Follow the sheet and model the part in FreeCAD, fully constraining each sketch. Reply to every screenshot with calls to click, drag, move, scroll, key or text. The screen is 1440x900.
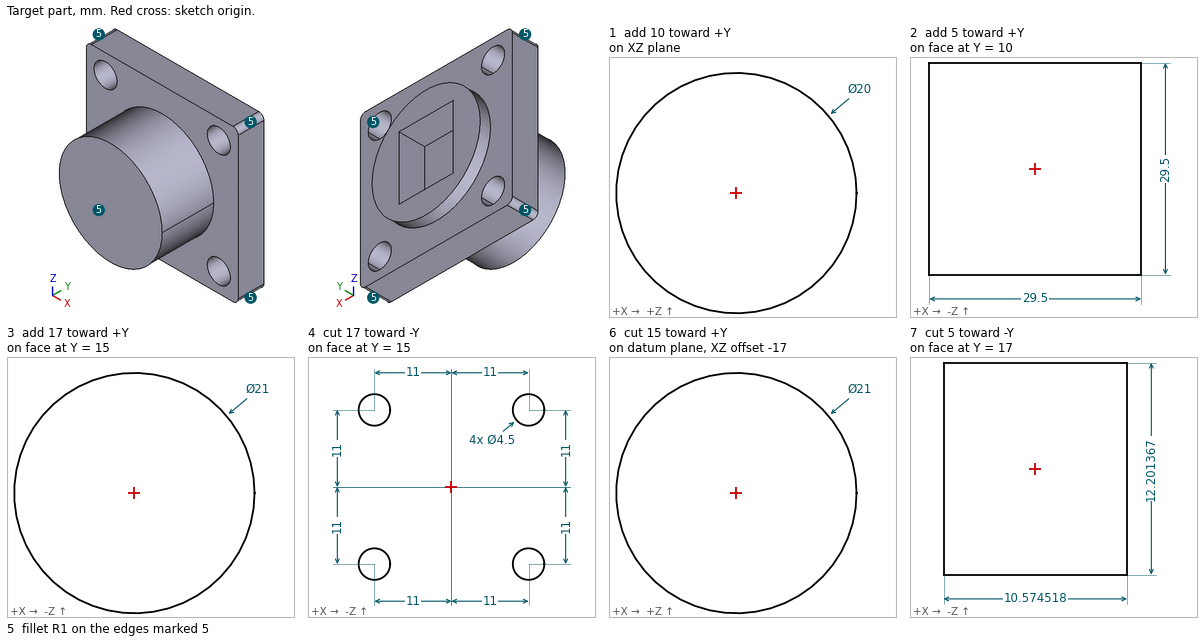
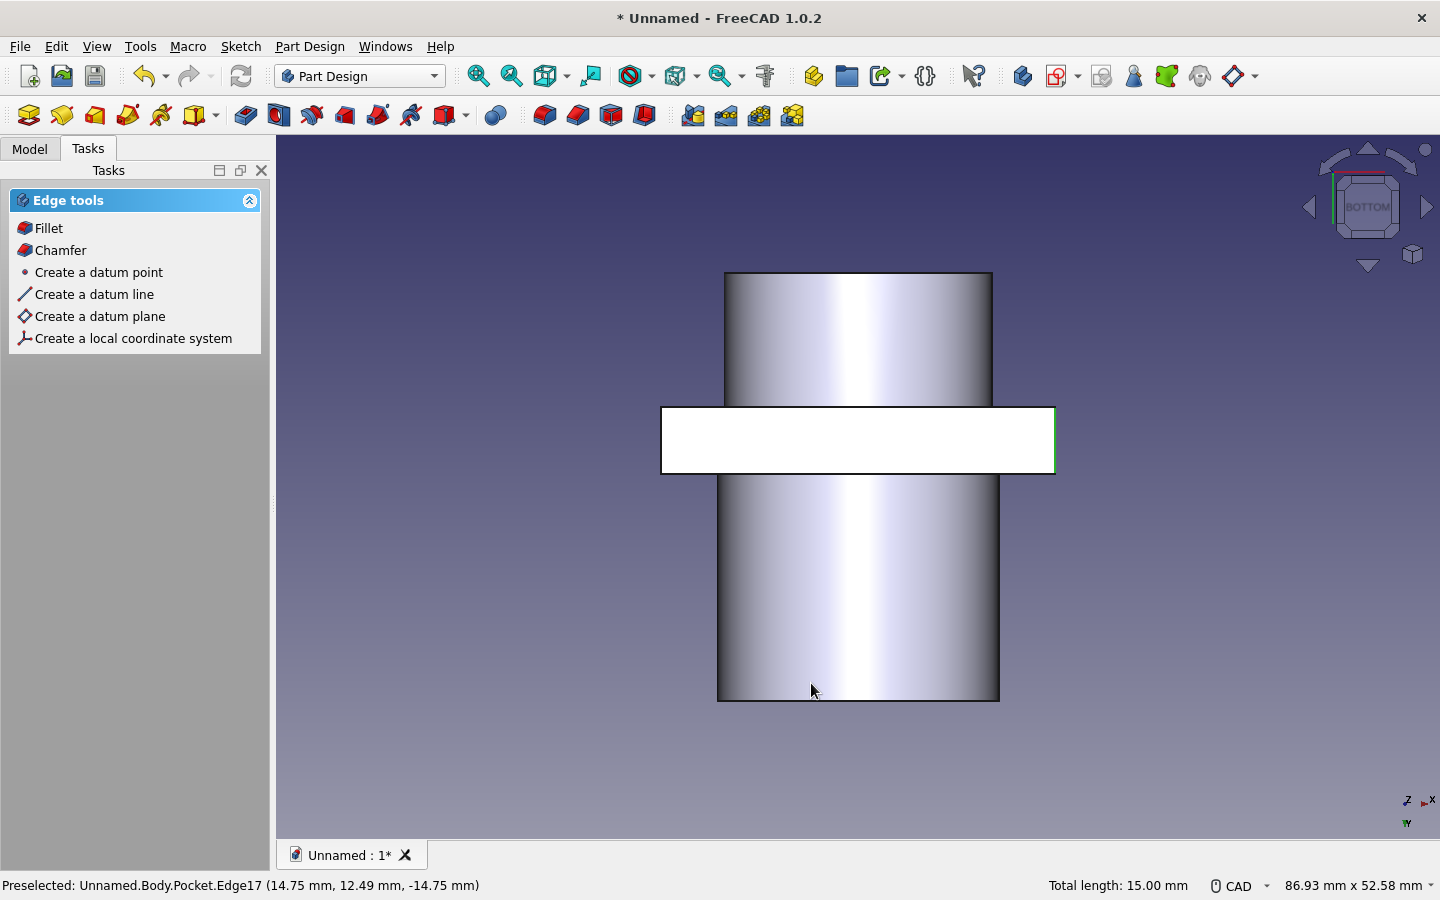
click(661, 439, ctrl)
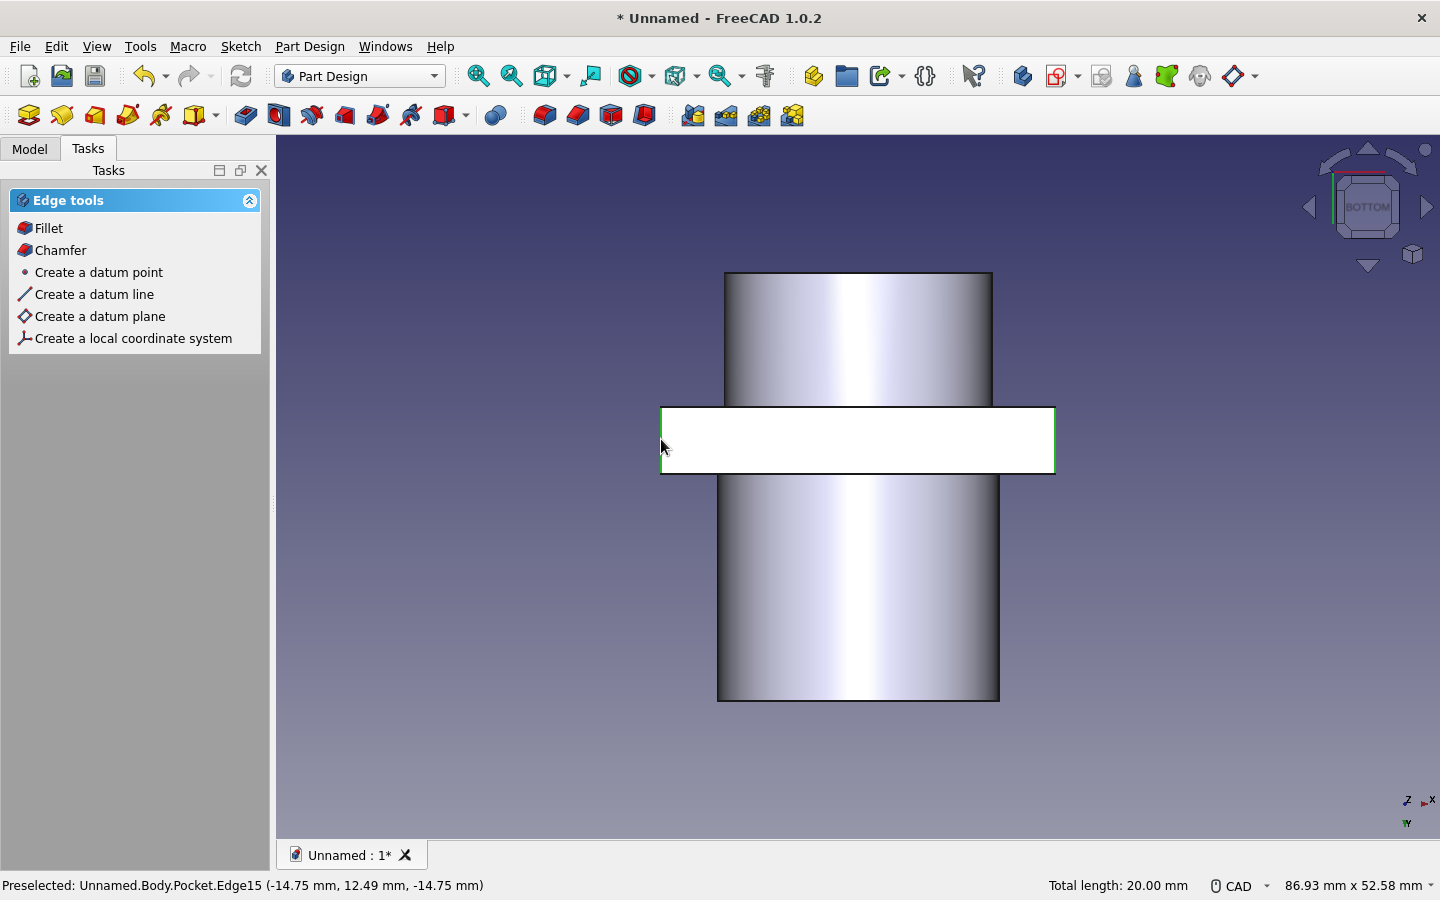
click(545, 116)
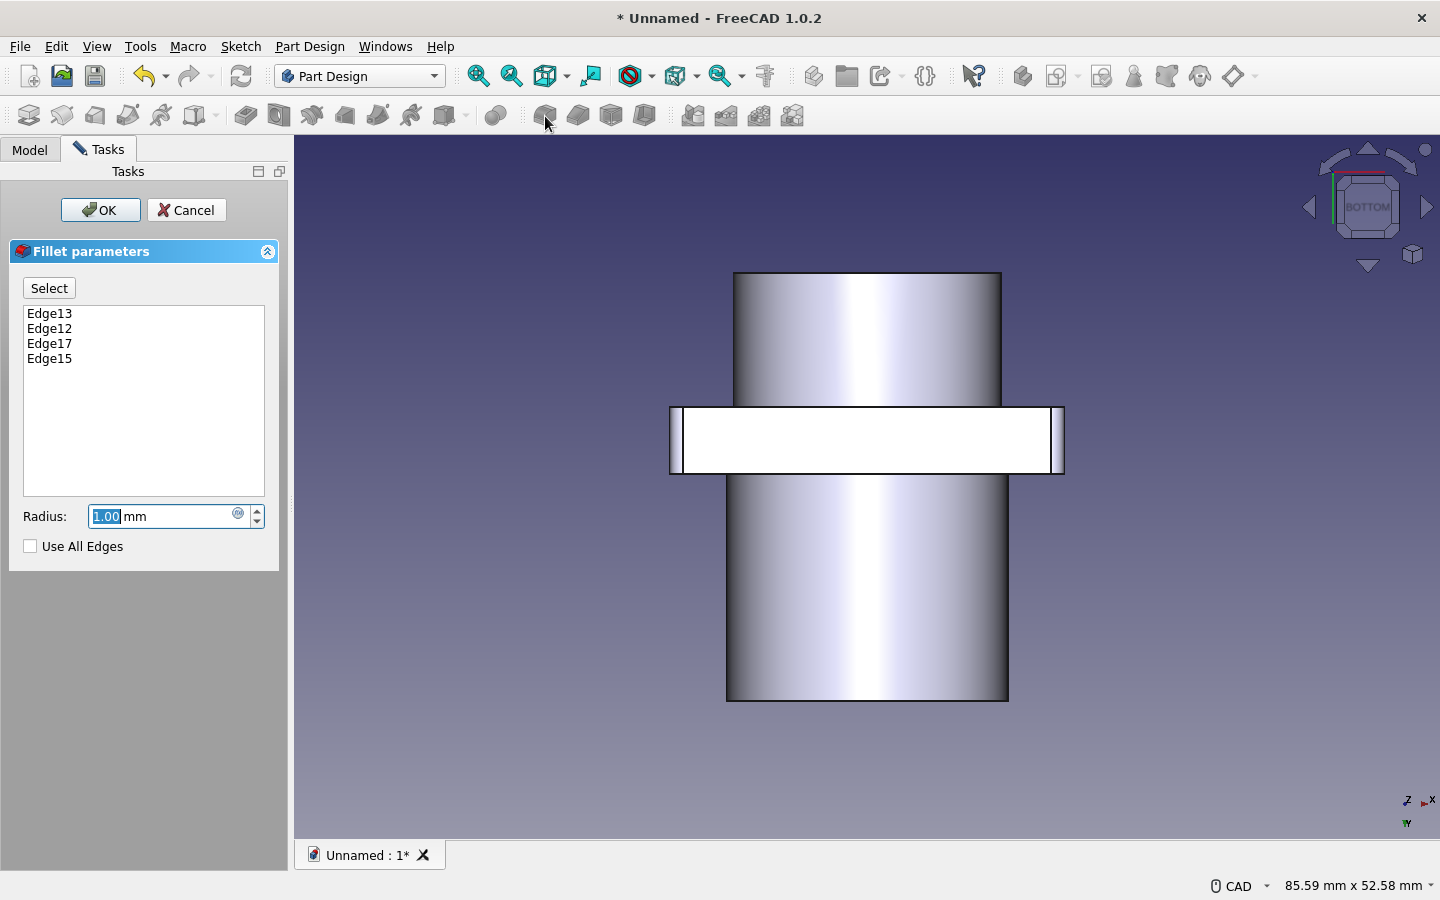
text(1)
key(Tab)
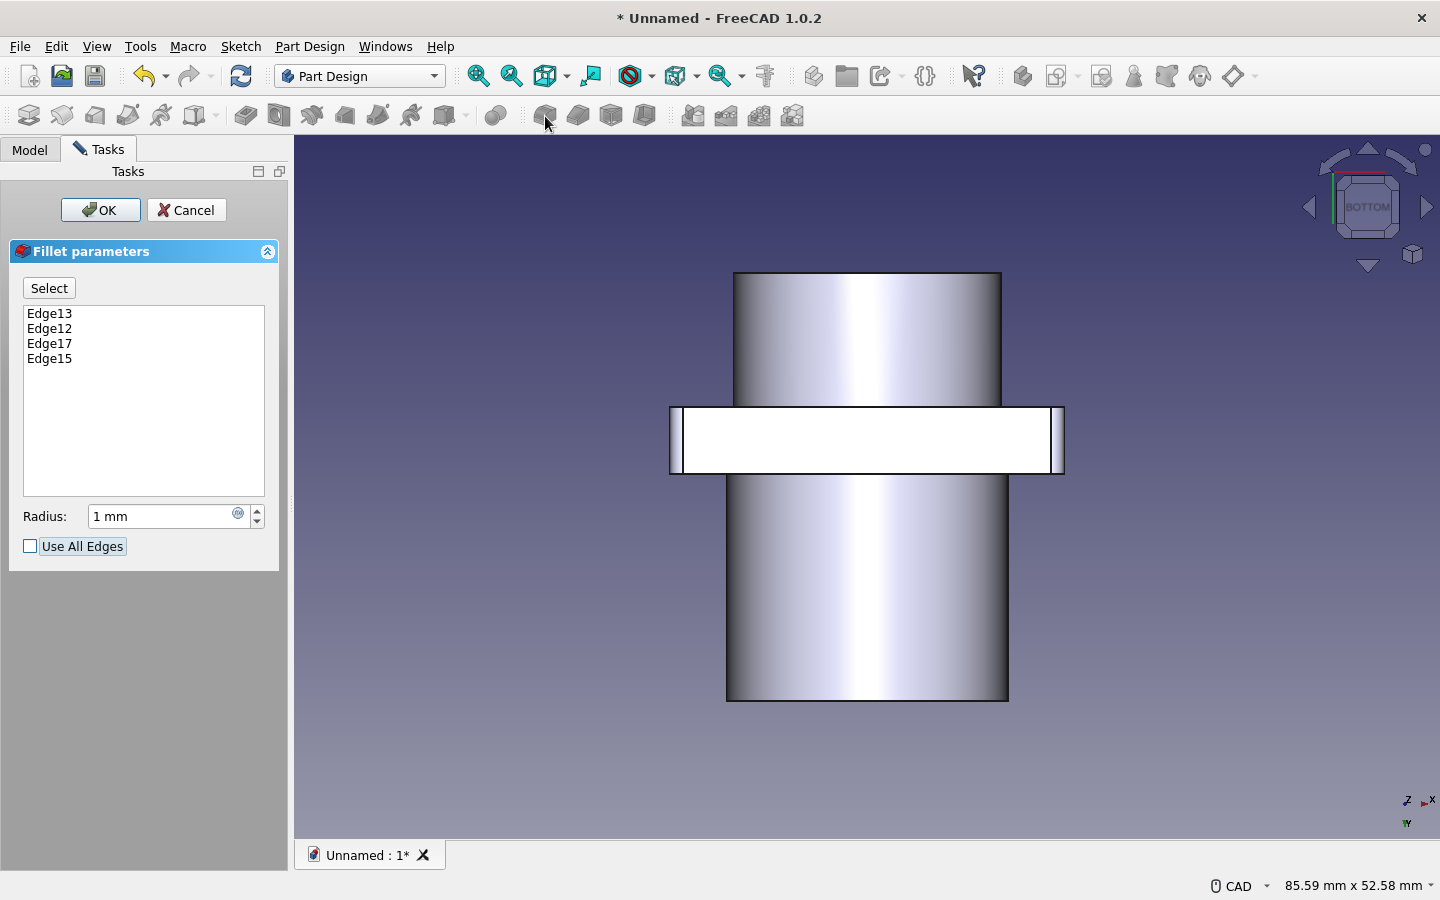
click(101, 210)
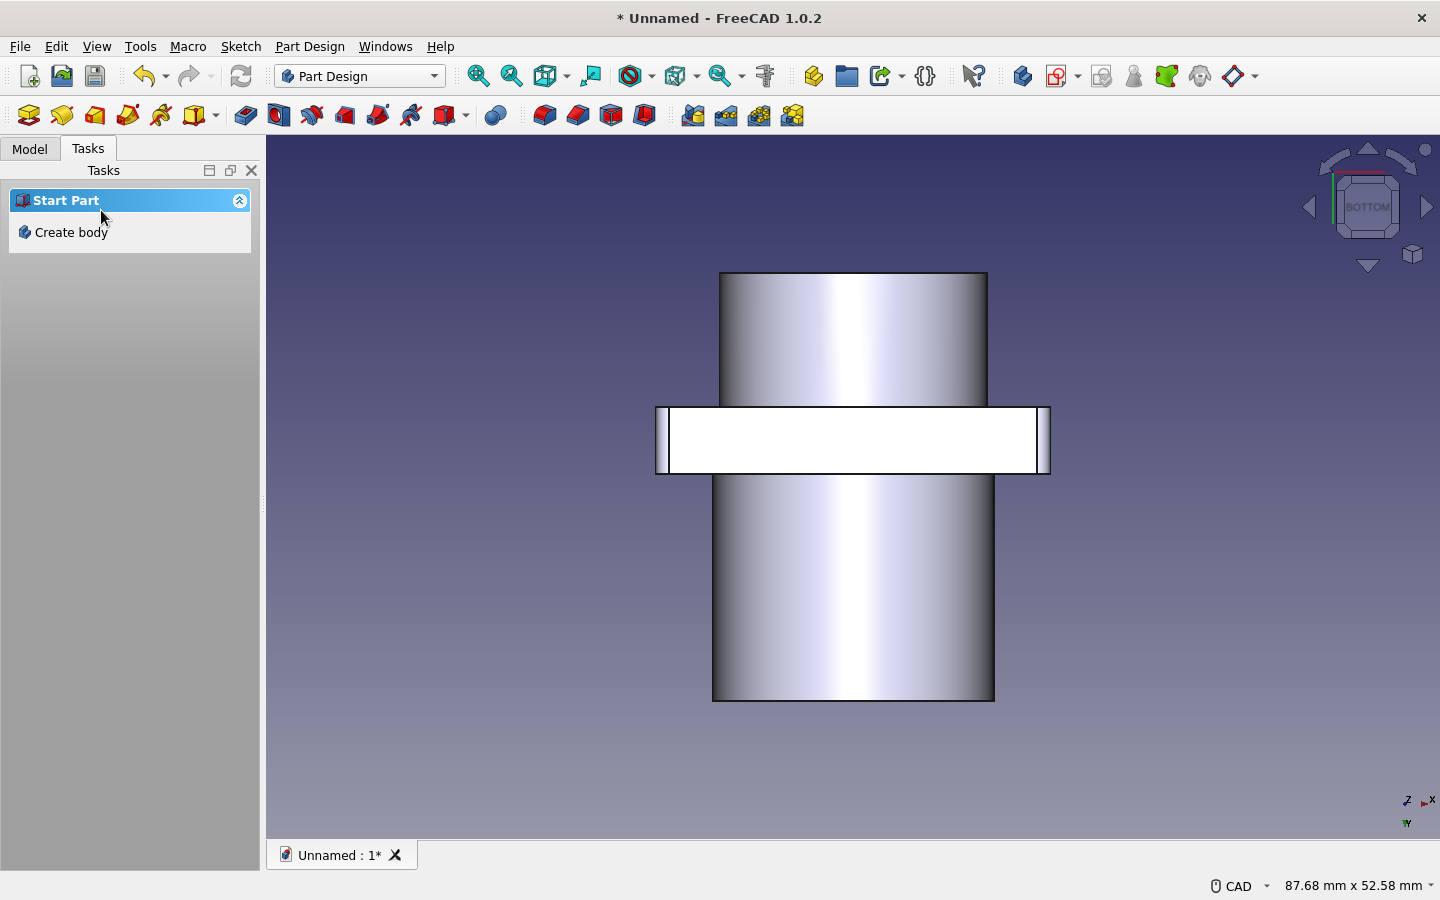
click(30, 148)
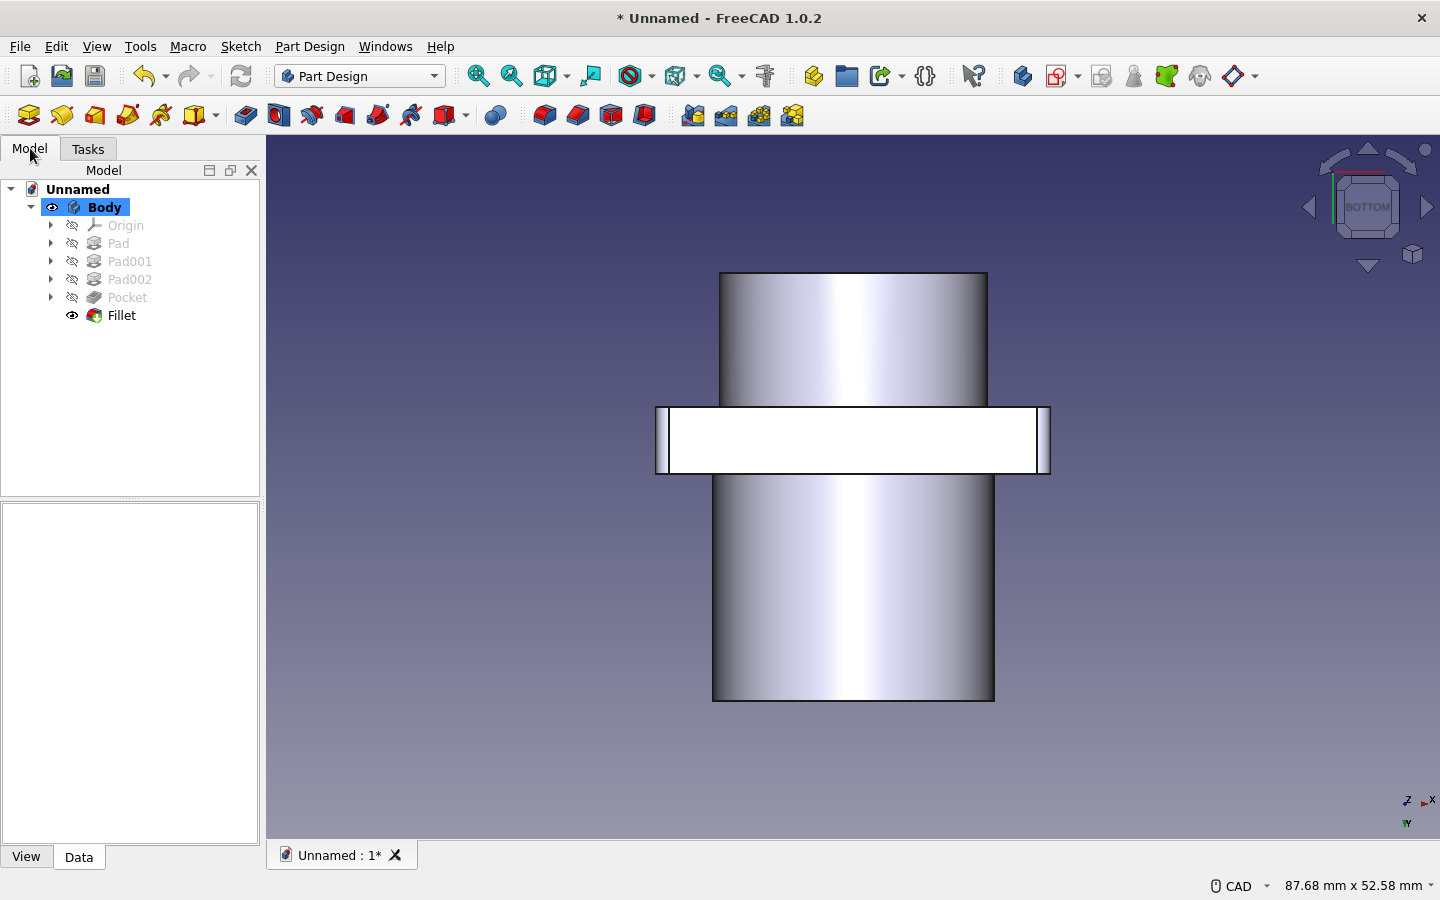
click(51, 225)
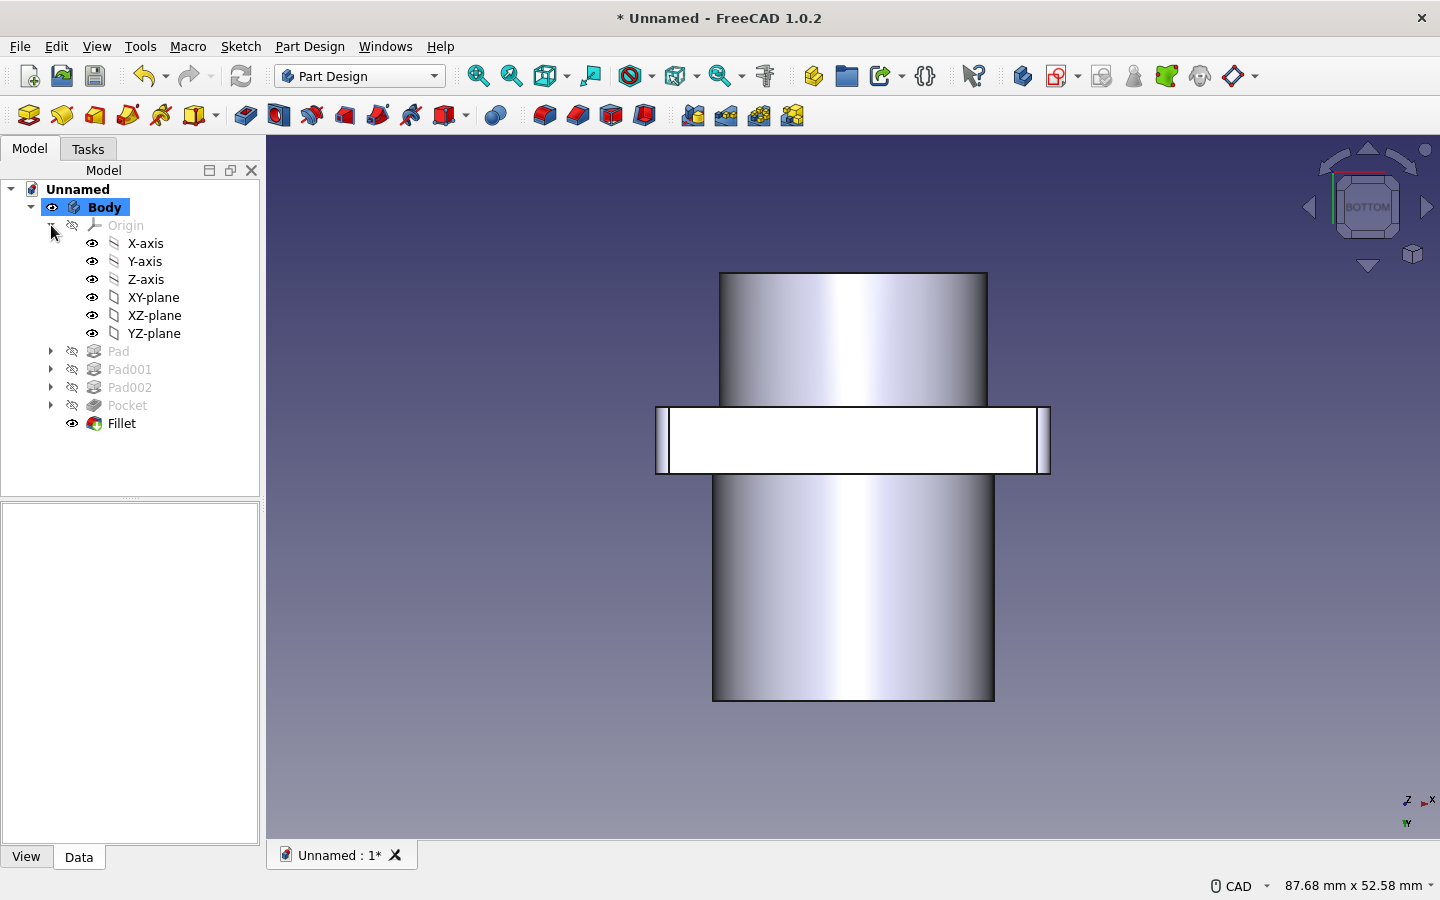
click(137, 315)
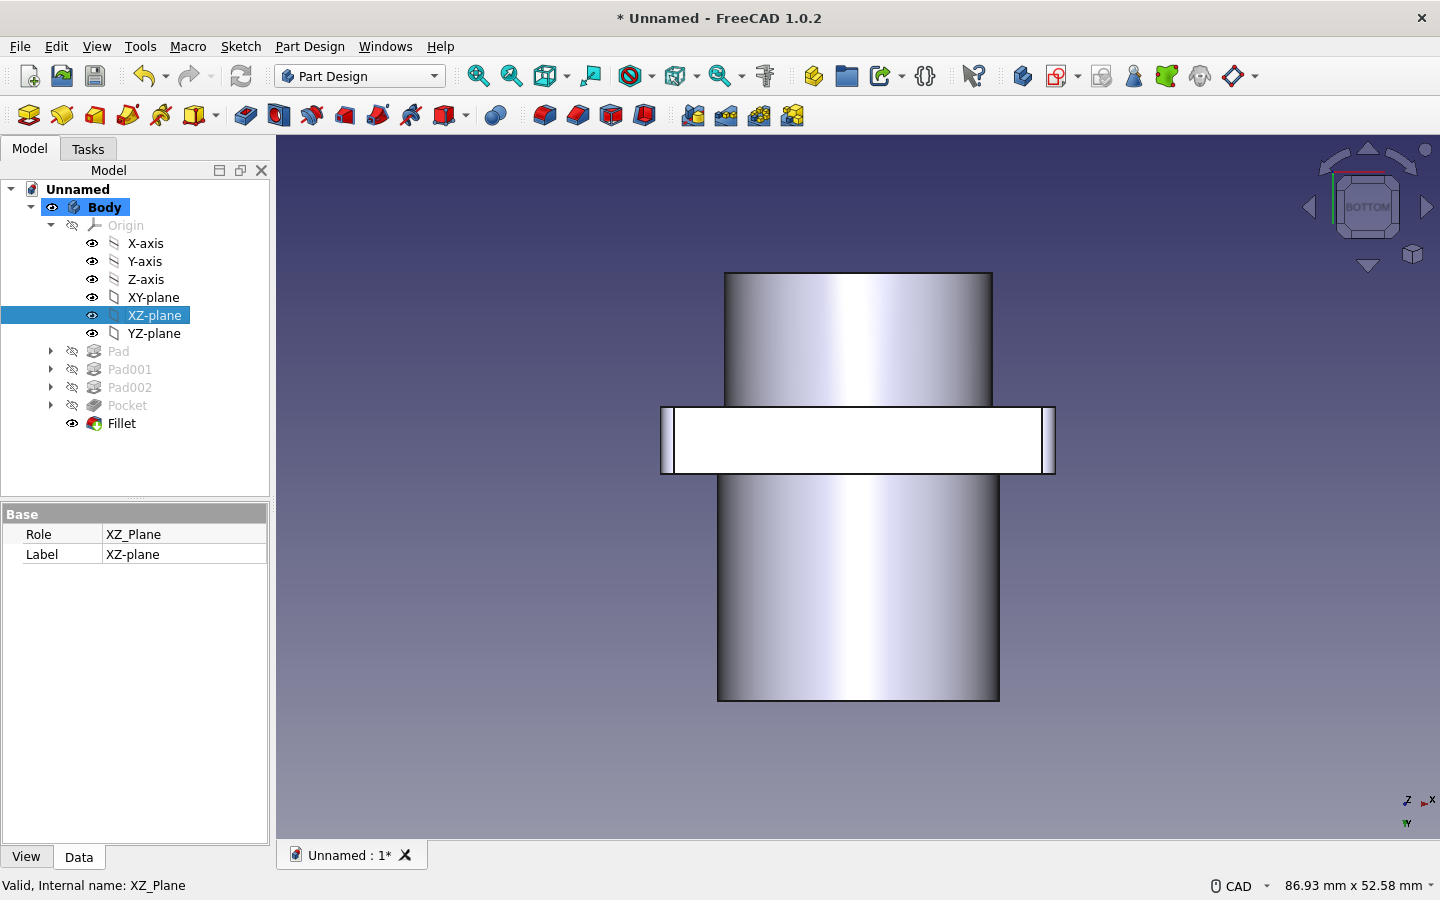
click(1232, 76)